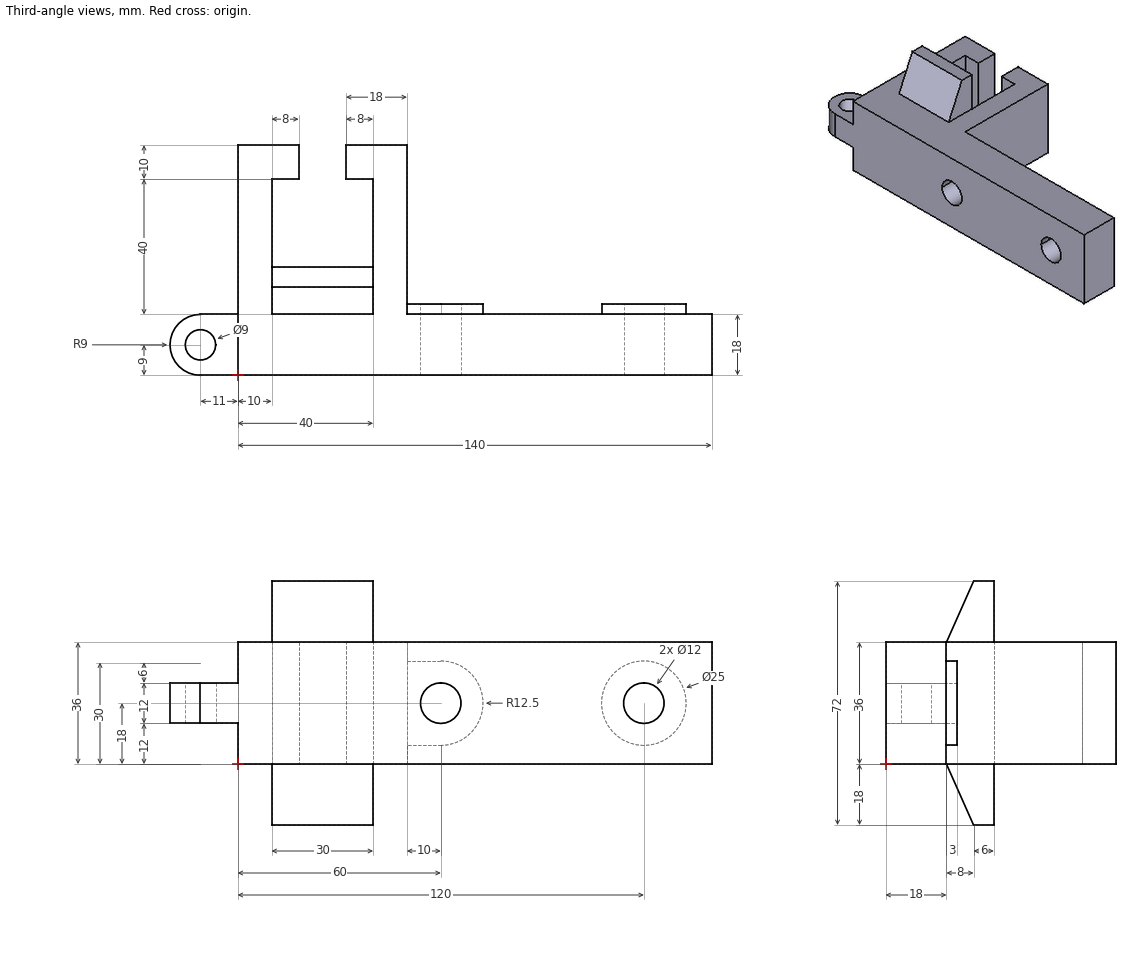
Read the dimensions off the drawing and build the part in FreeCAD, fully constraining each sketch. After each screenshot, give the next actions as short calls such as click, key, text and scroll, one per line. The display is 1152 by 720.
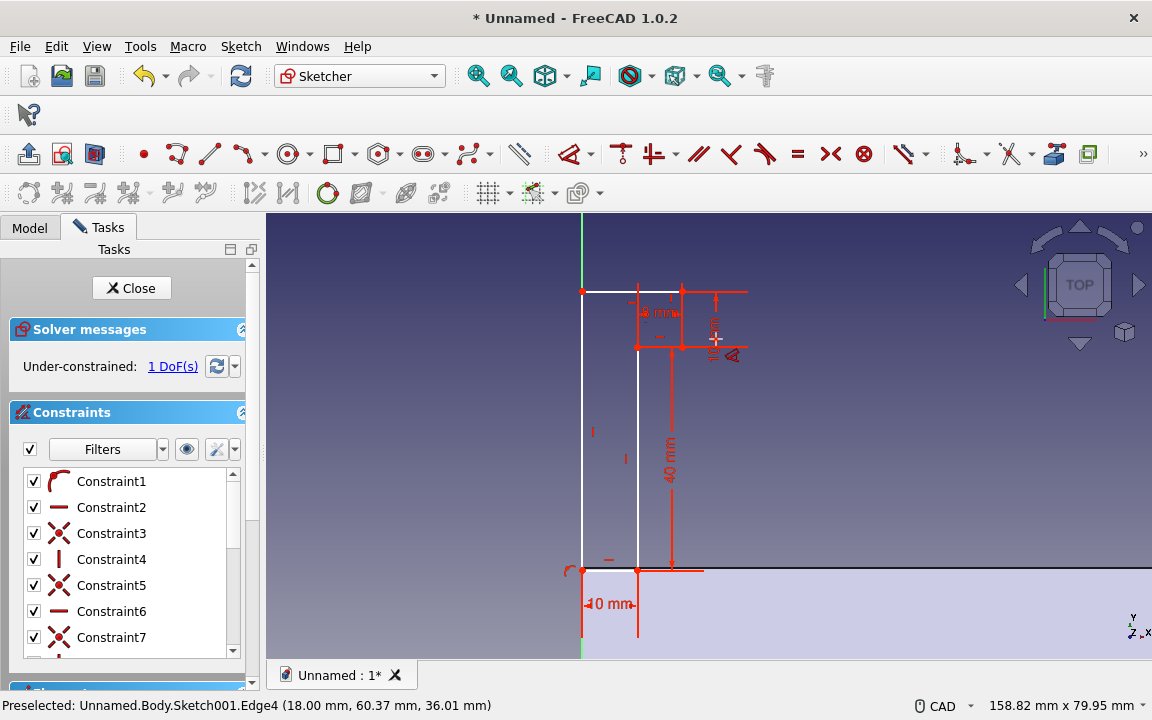
click(582, 571)
click(548, 580)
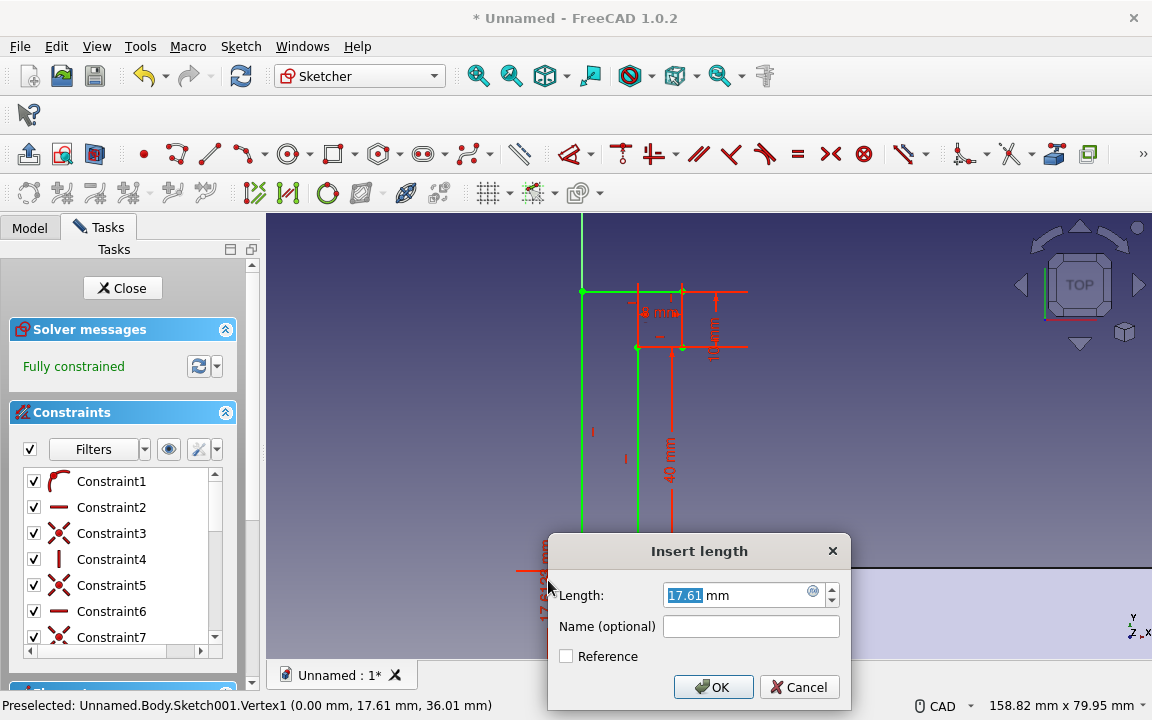
text(18)
key(Return)
key(Escape)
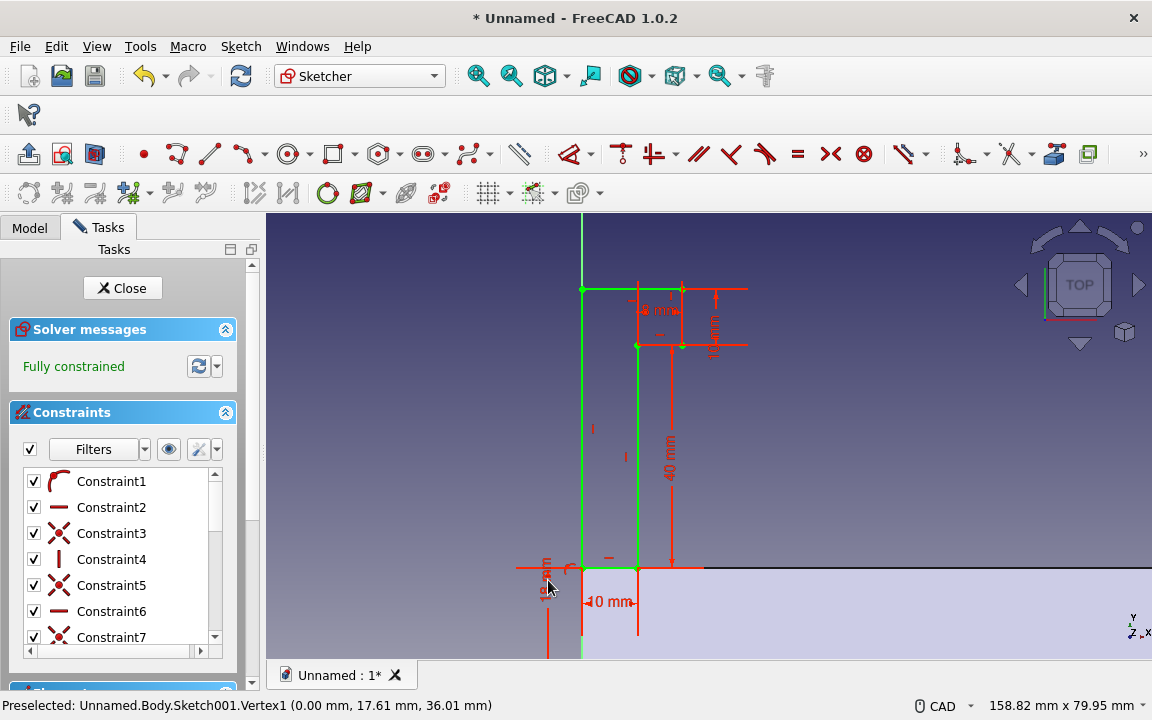
click(123, 288)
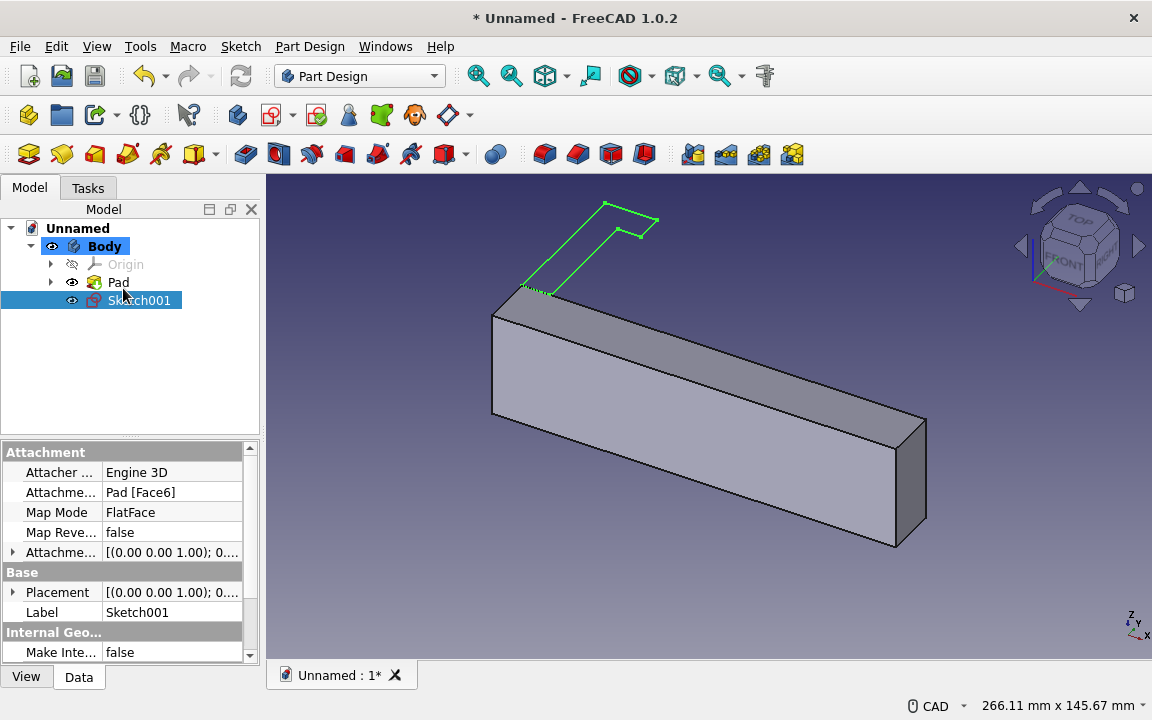
click(29, 154)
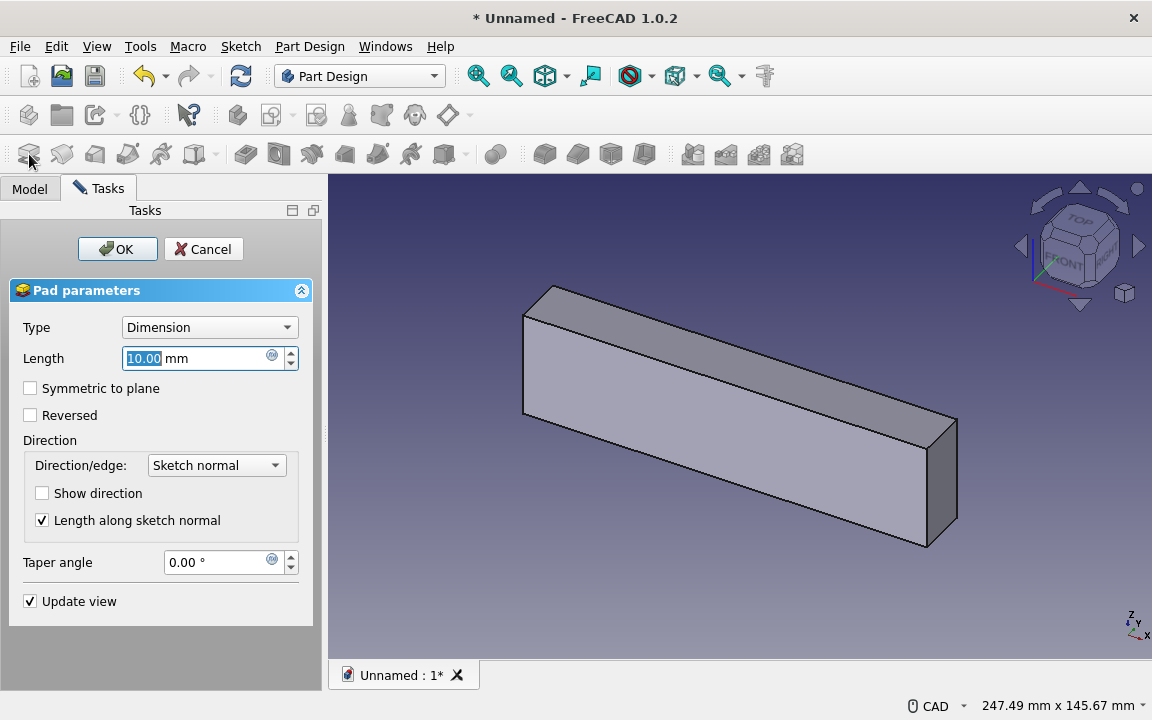
text(36)
key(Tab)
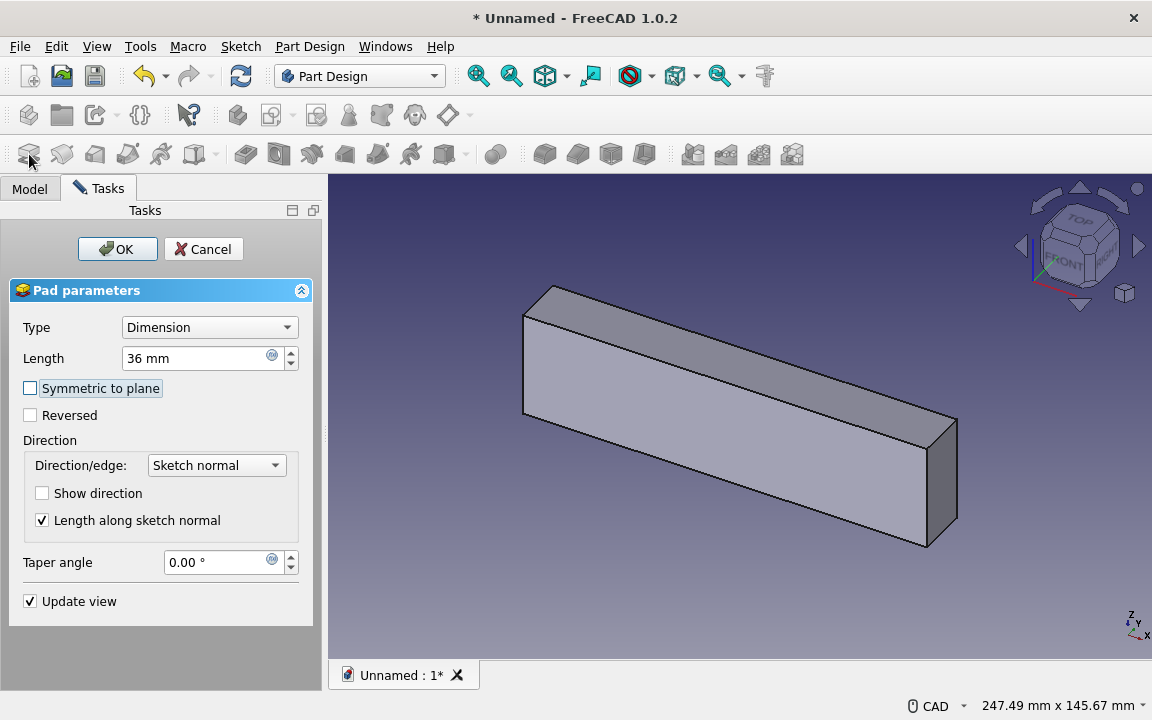
click(31, 415)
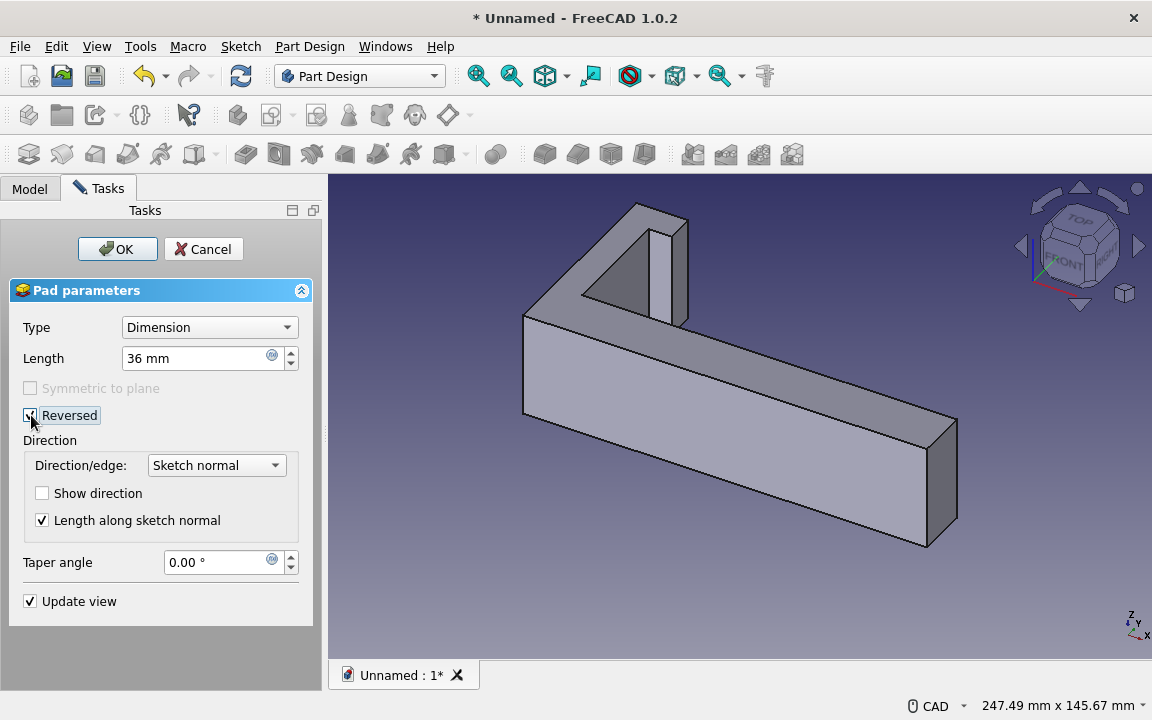
click(118, 249)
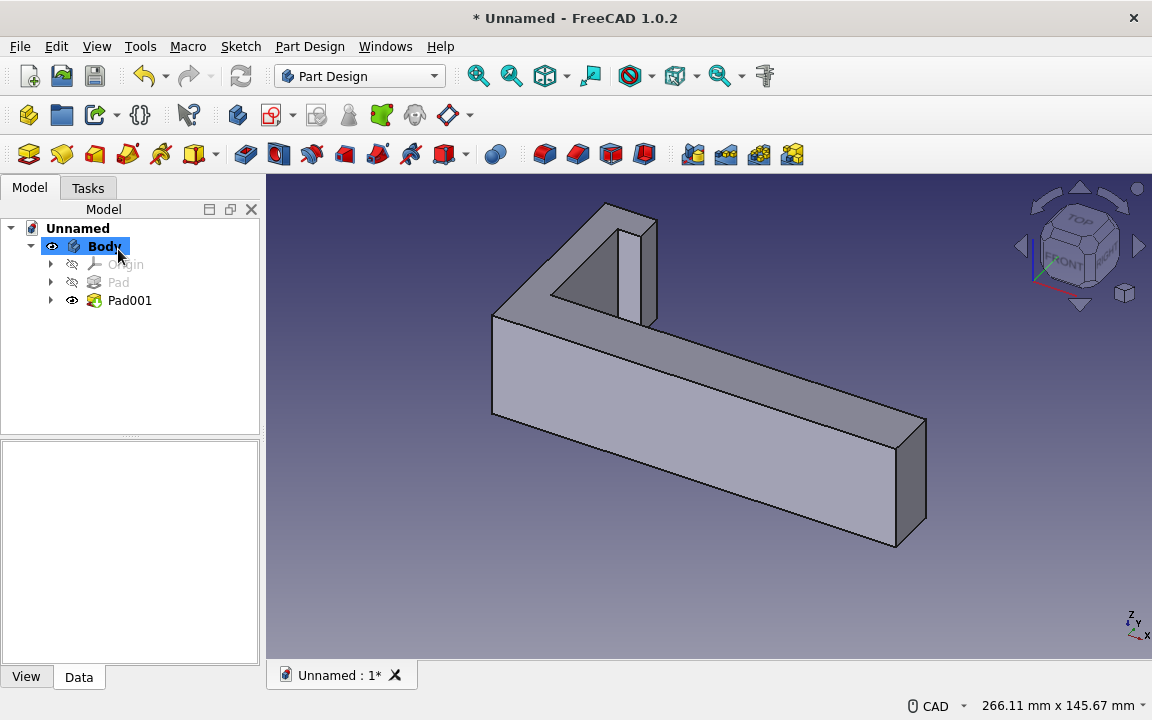
click(594, 287)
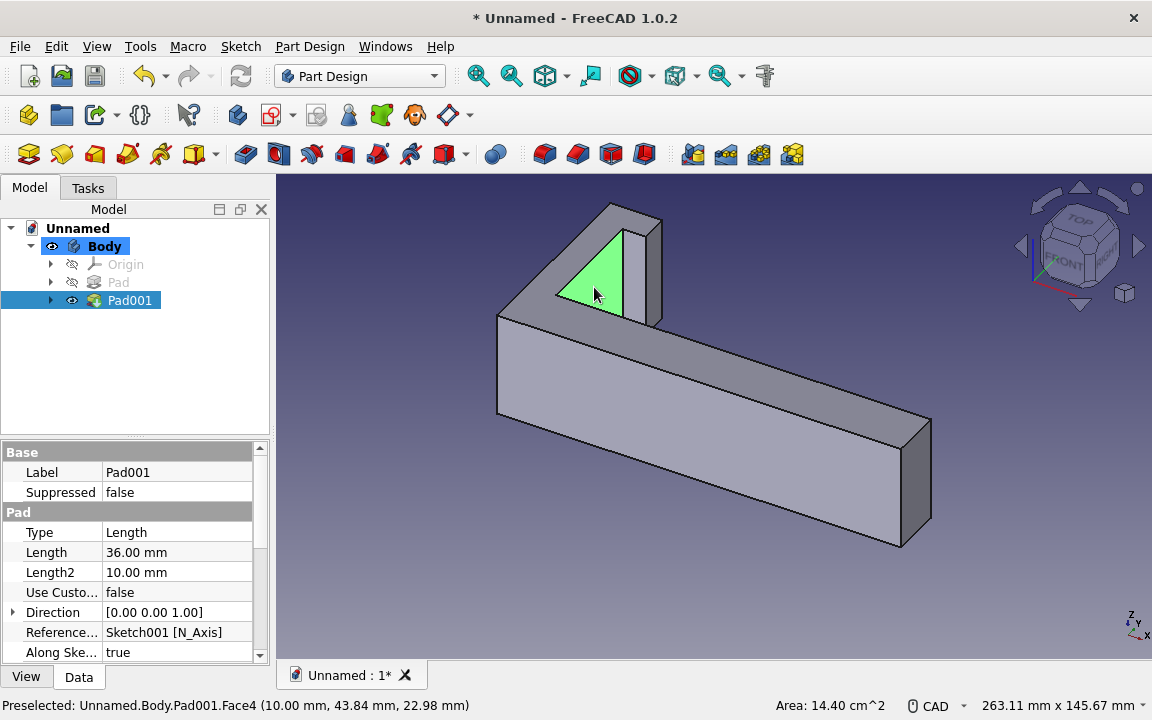
click(270, 116)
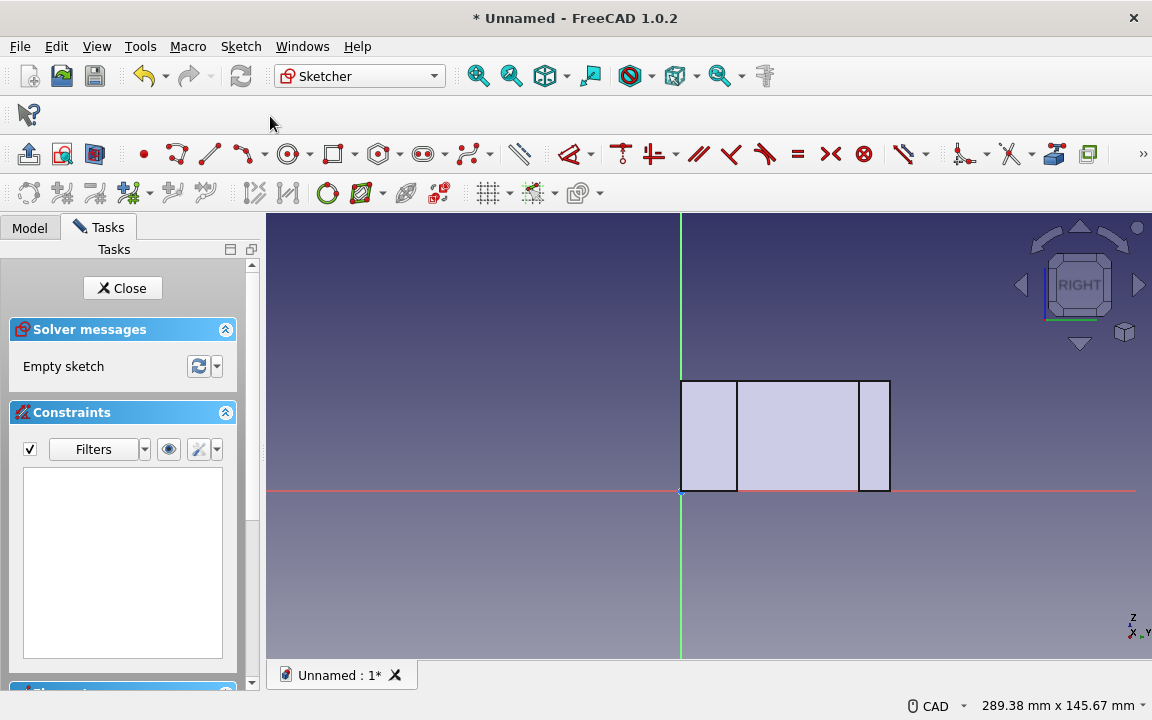
key(g)
key(m)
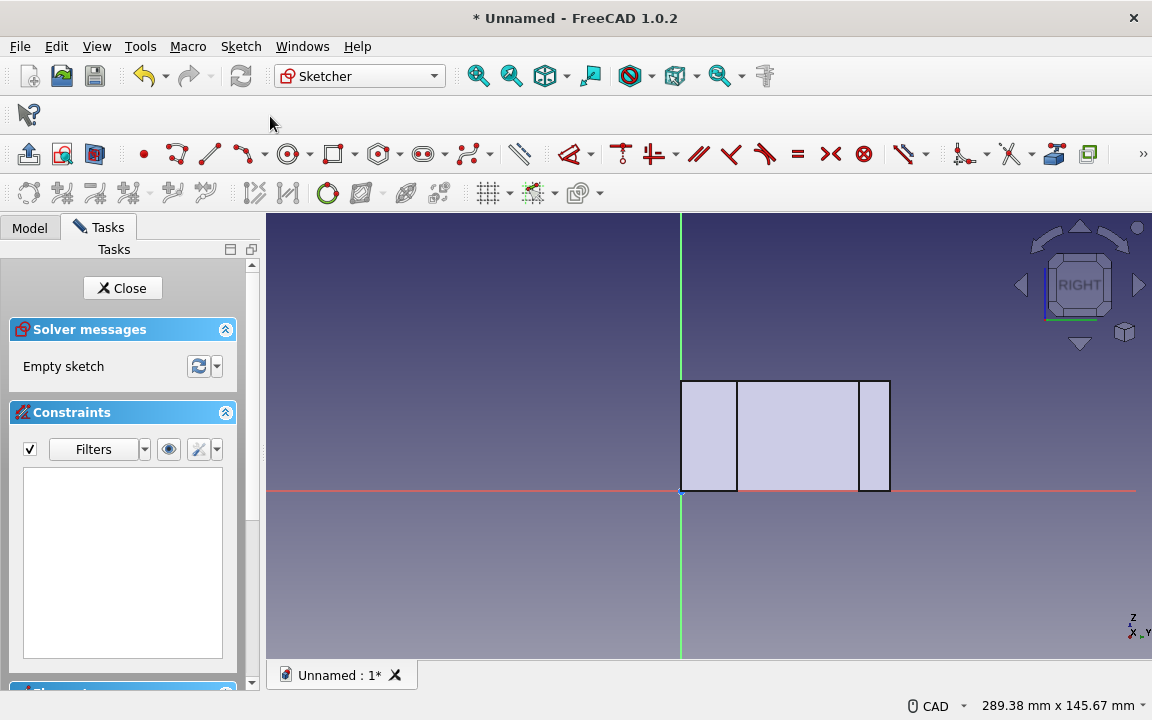
click(737, 491)
click(761, 546)
click(779, 546)
click(779, 326)
click(761, 326)
click(737, 381)
click(737, 491)
key(Escape)
key(Escape)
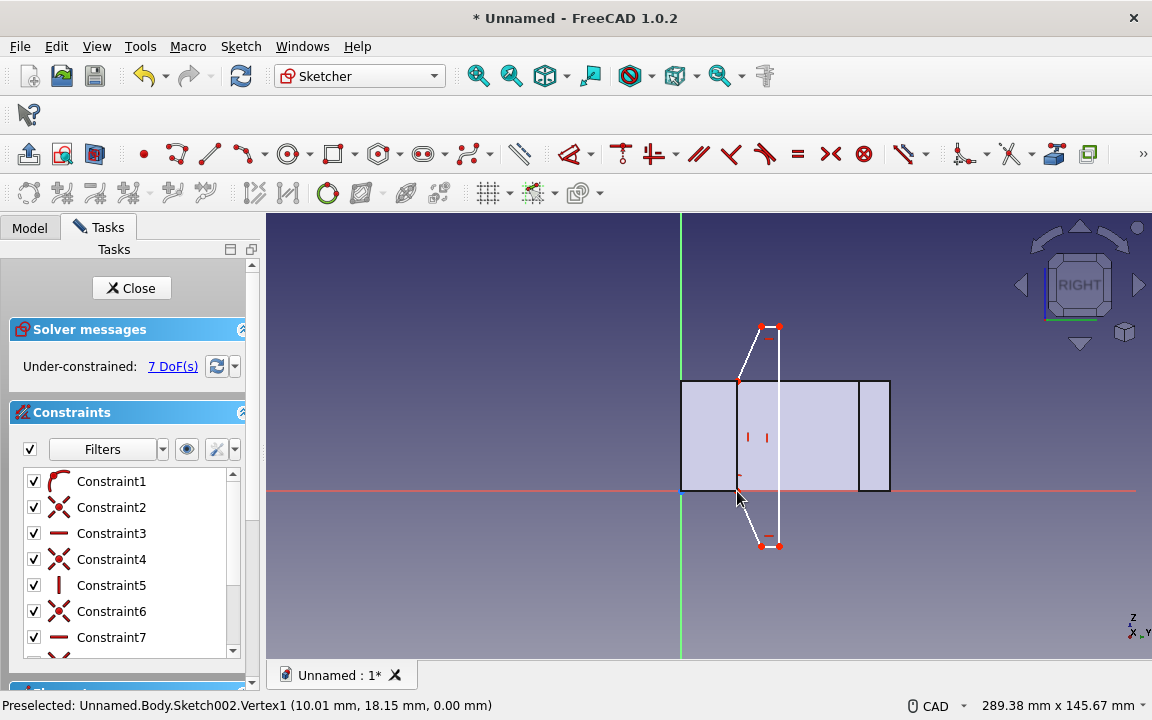
key(d)